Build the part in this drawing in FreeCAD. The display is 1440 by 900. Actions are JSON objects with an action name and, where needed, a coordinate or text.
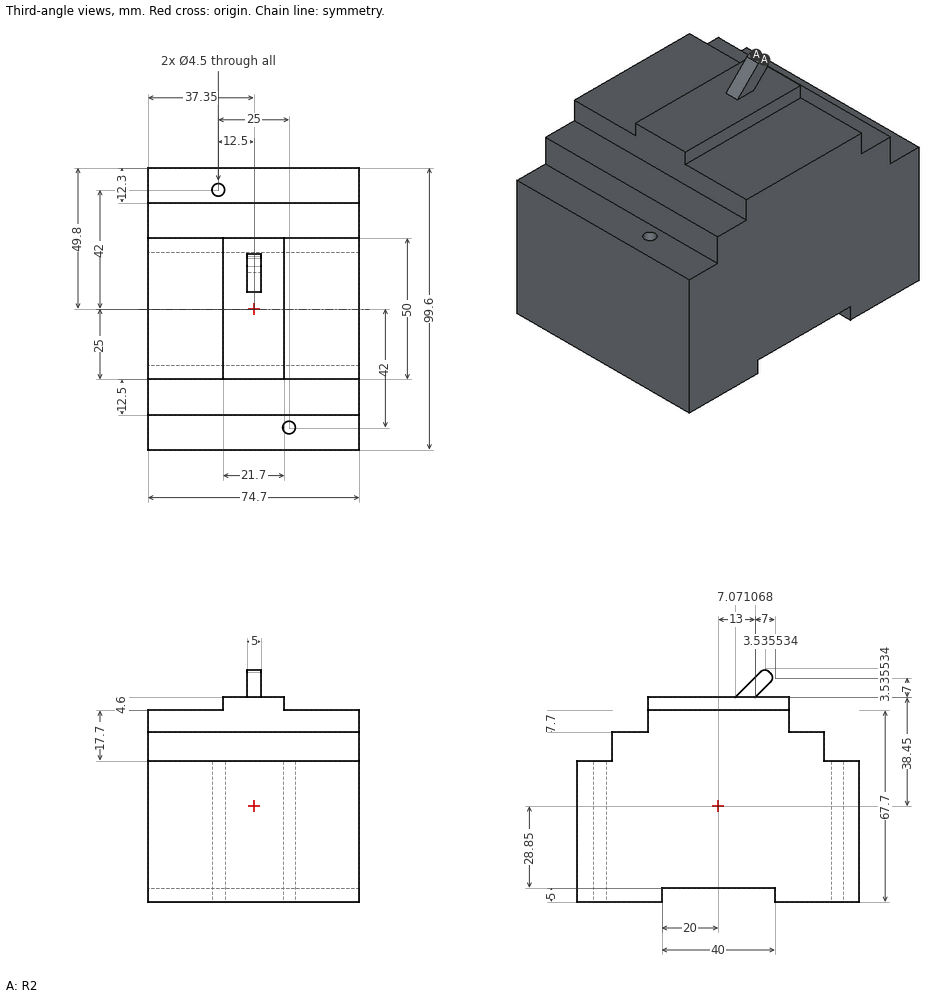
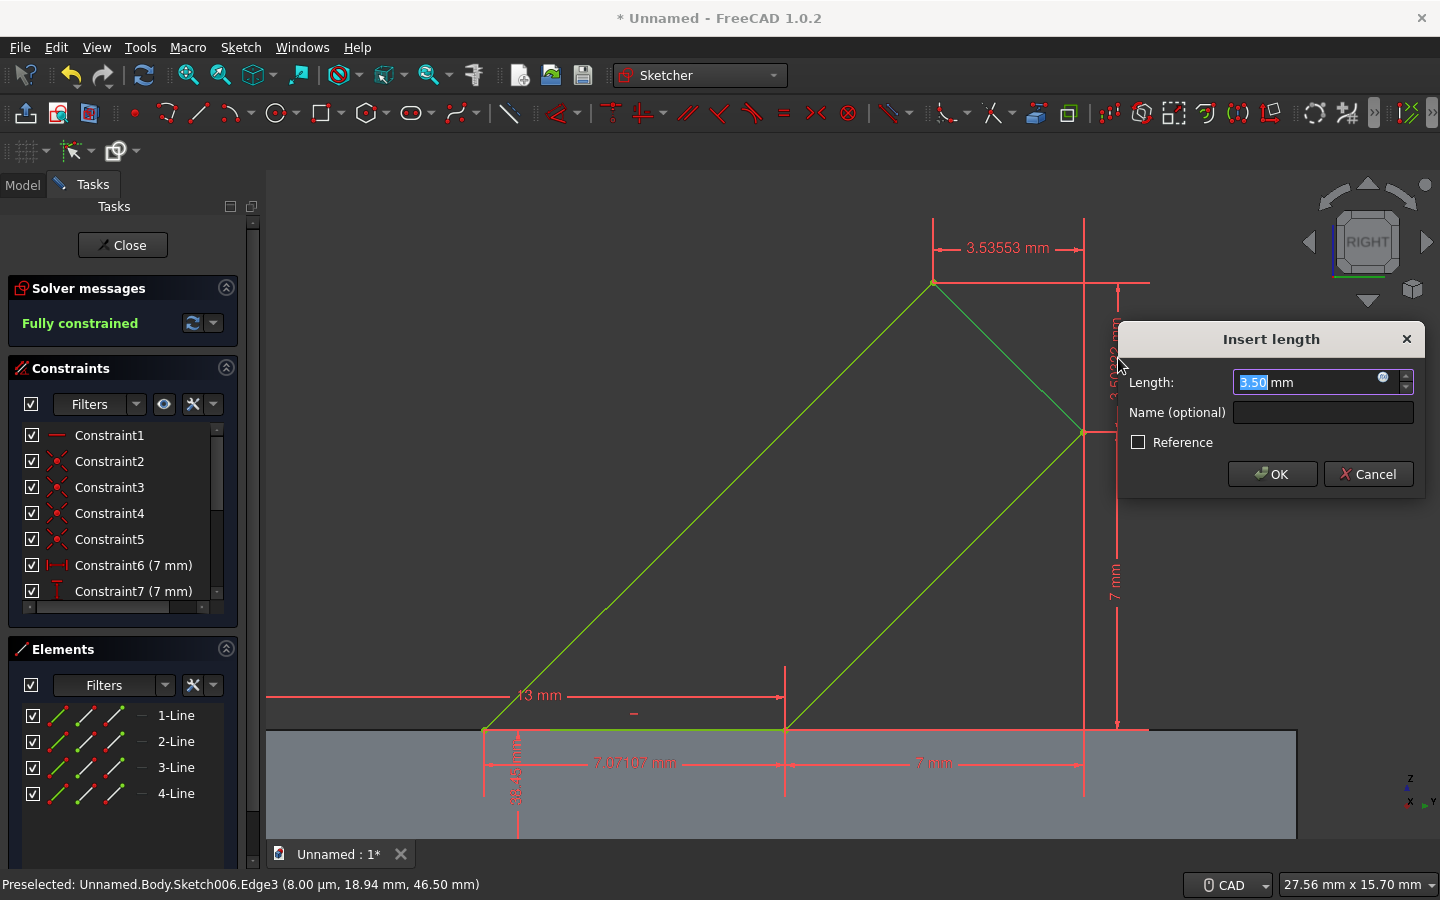
{"action": "type", "text": "3.535534"}
{"action": "key", "text": "Return"}
{"action": "key", "text": "Escape"}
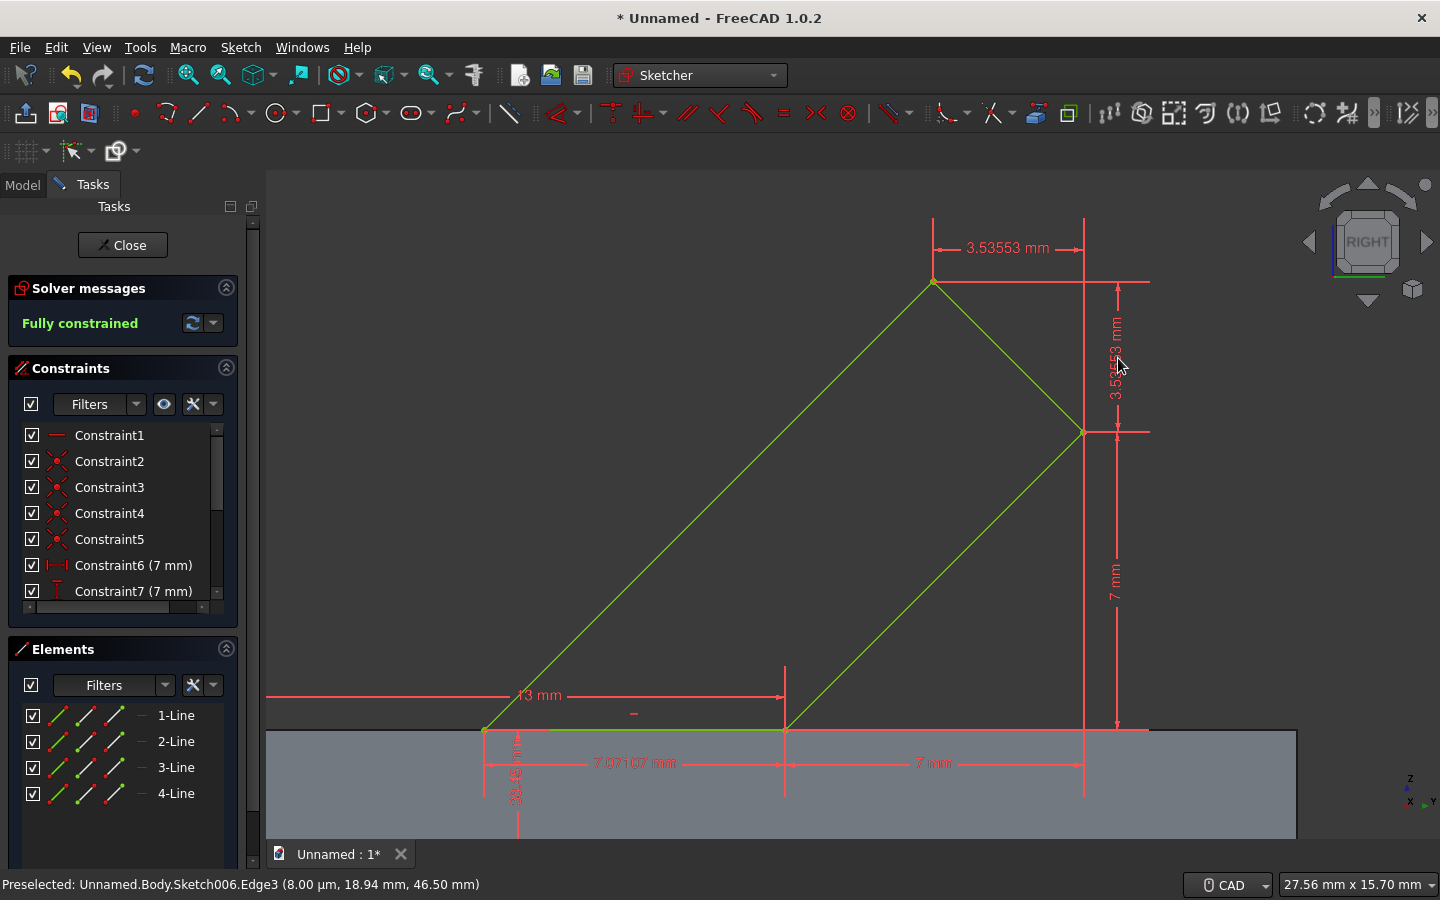
{"action": "left_click", "coordinate": [123, 245]}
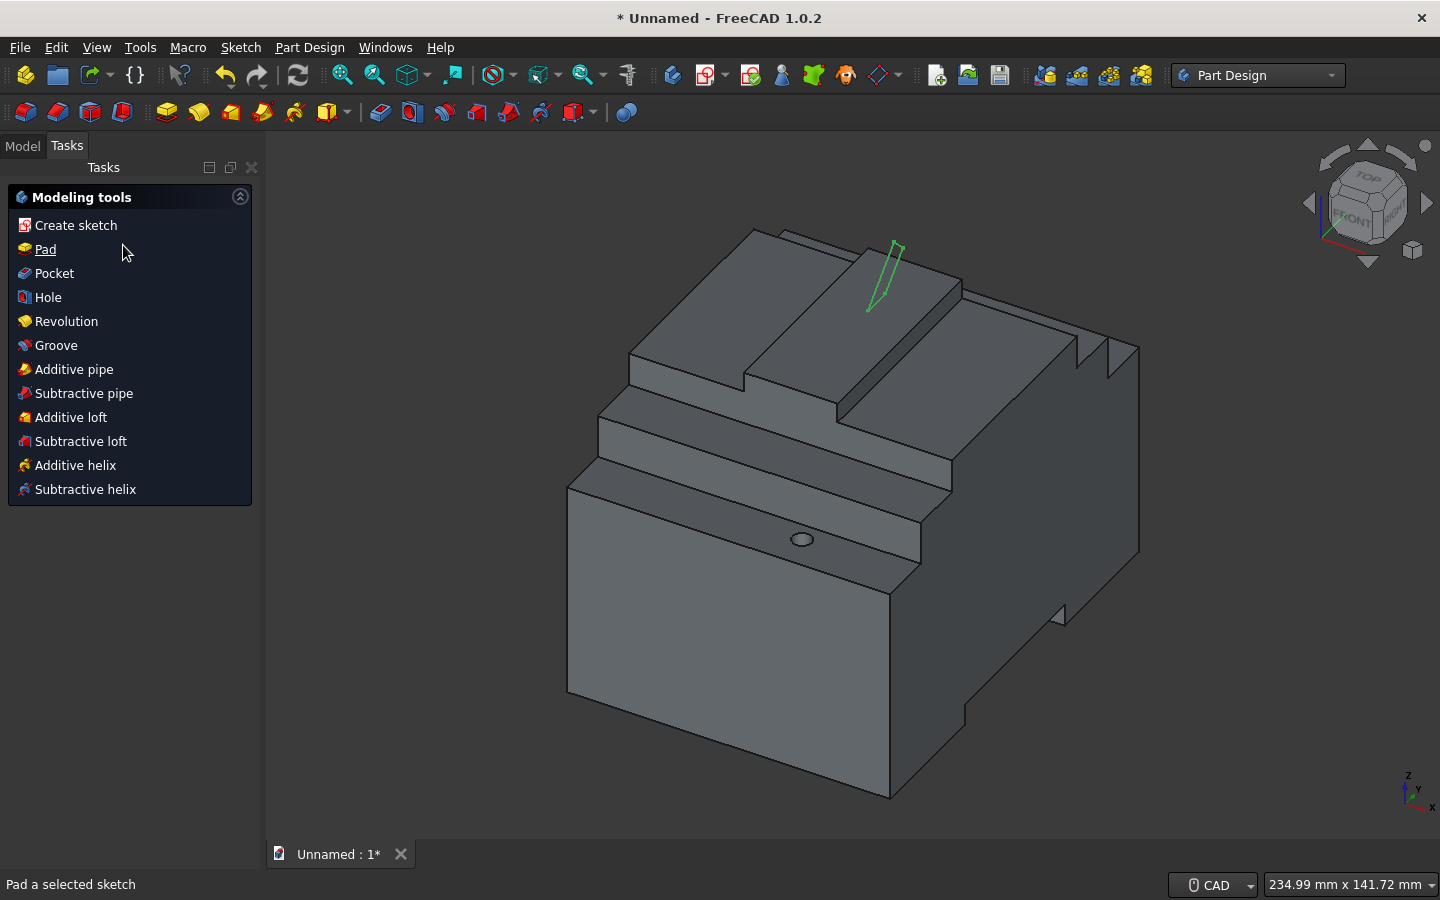
{"action": "left_click", "coordinate": [168, 112]}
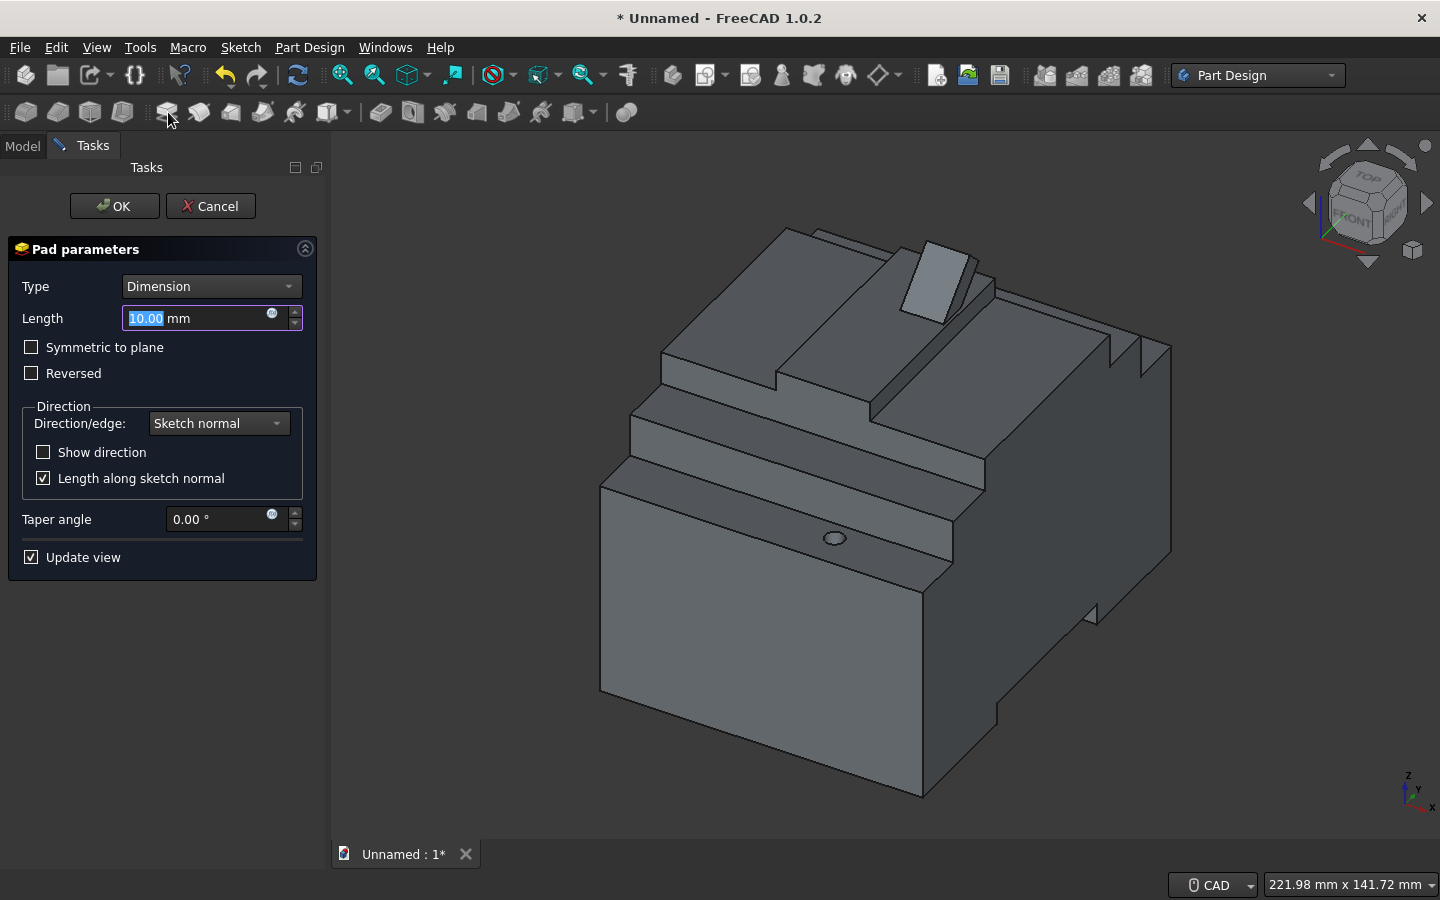
{"action": "type", "text": "5"}
{"action": "key", "text": "Tab"}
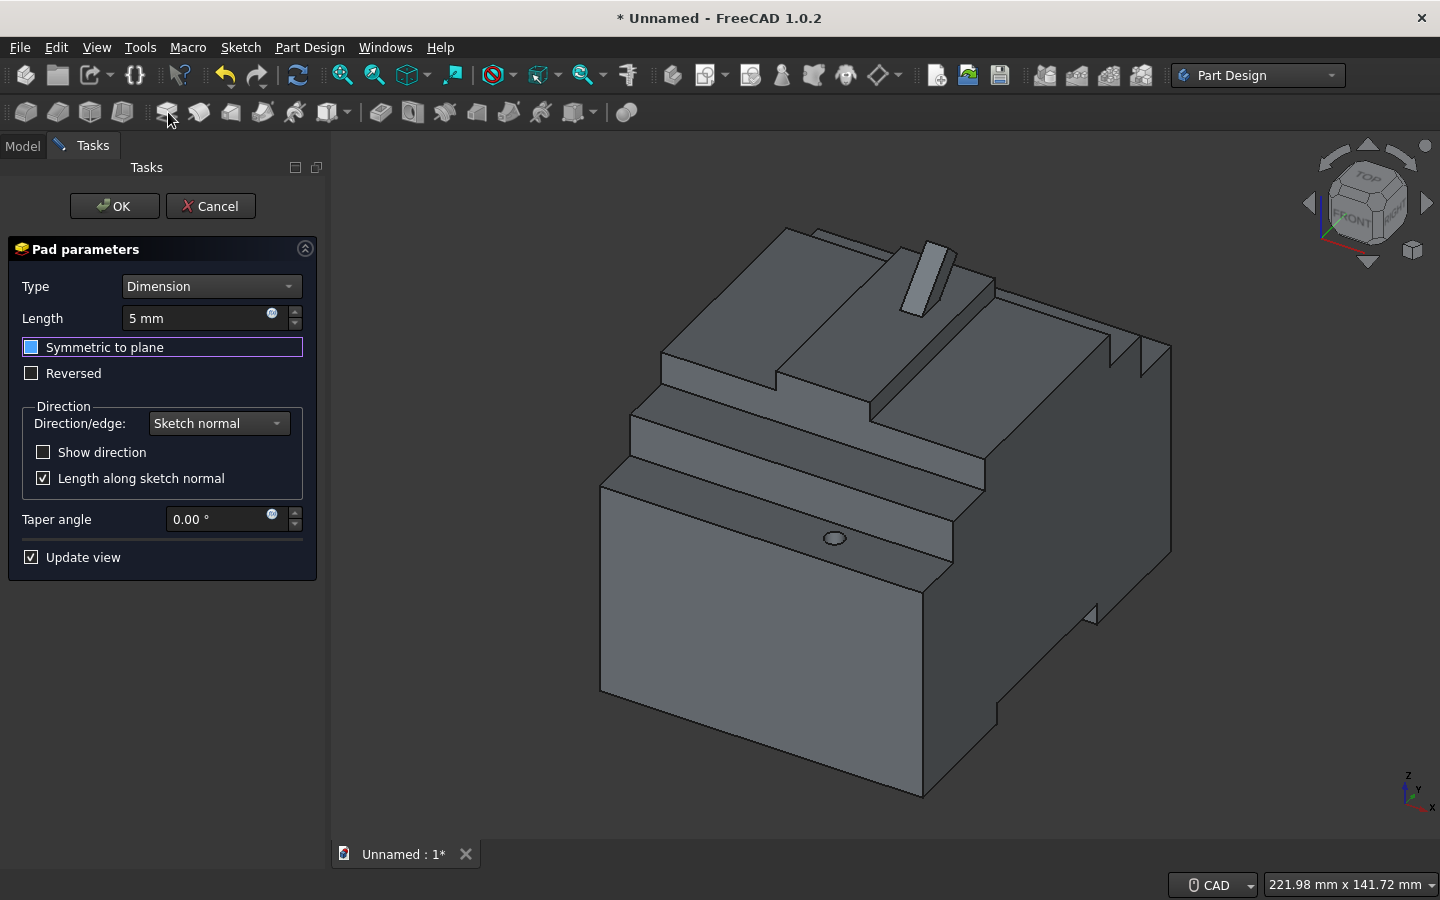
{"action": "left_click", "coordinate": [30, 347]}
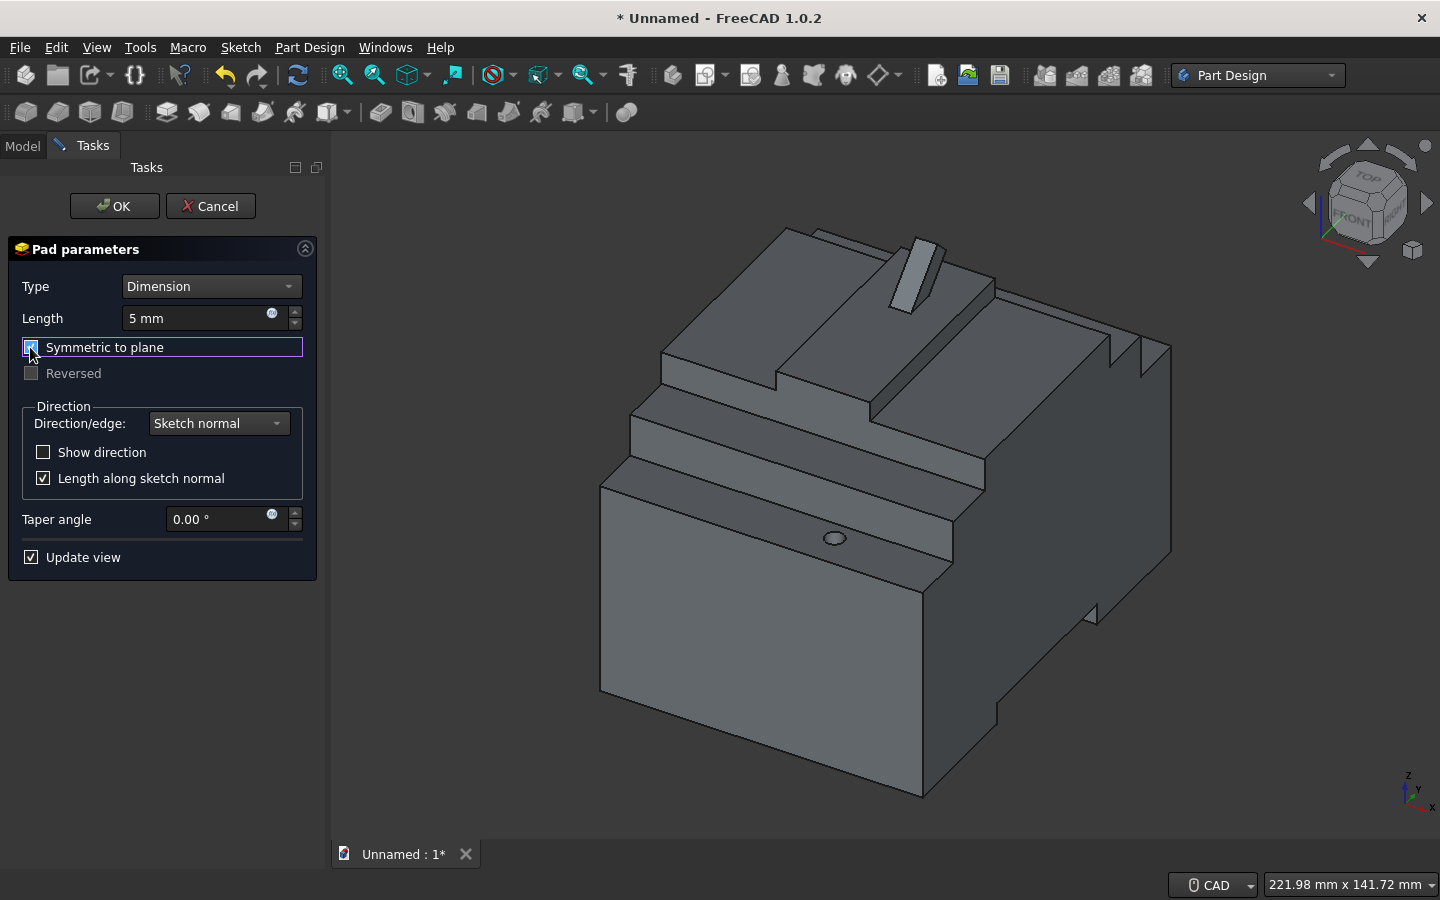
{"action": "left_click", "coordinate": [115, 206]}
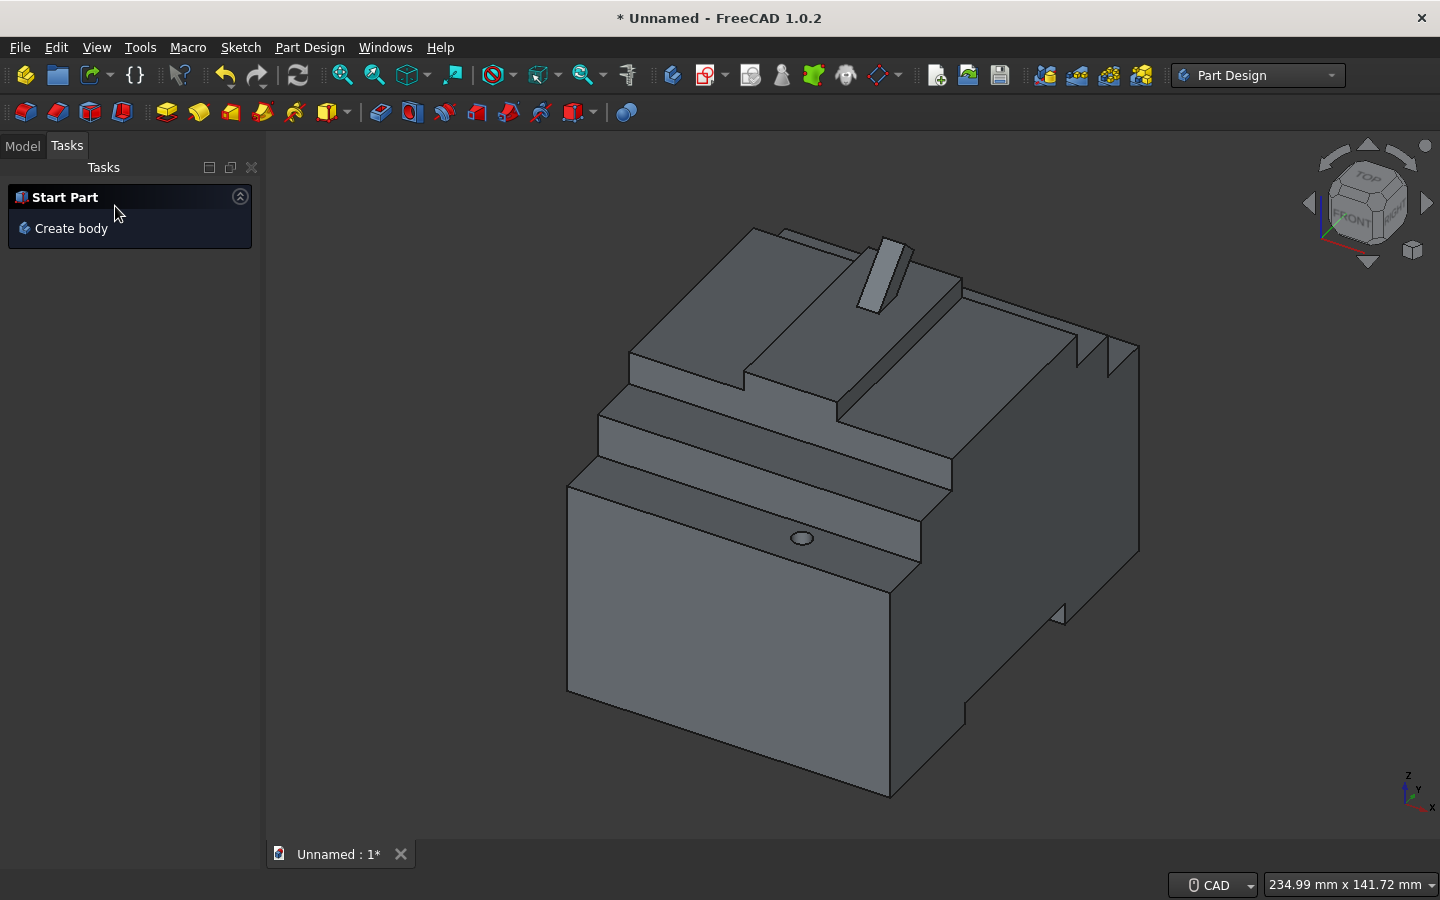
{"action": "key", "text": "v f"}